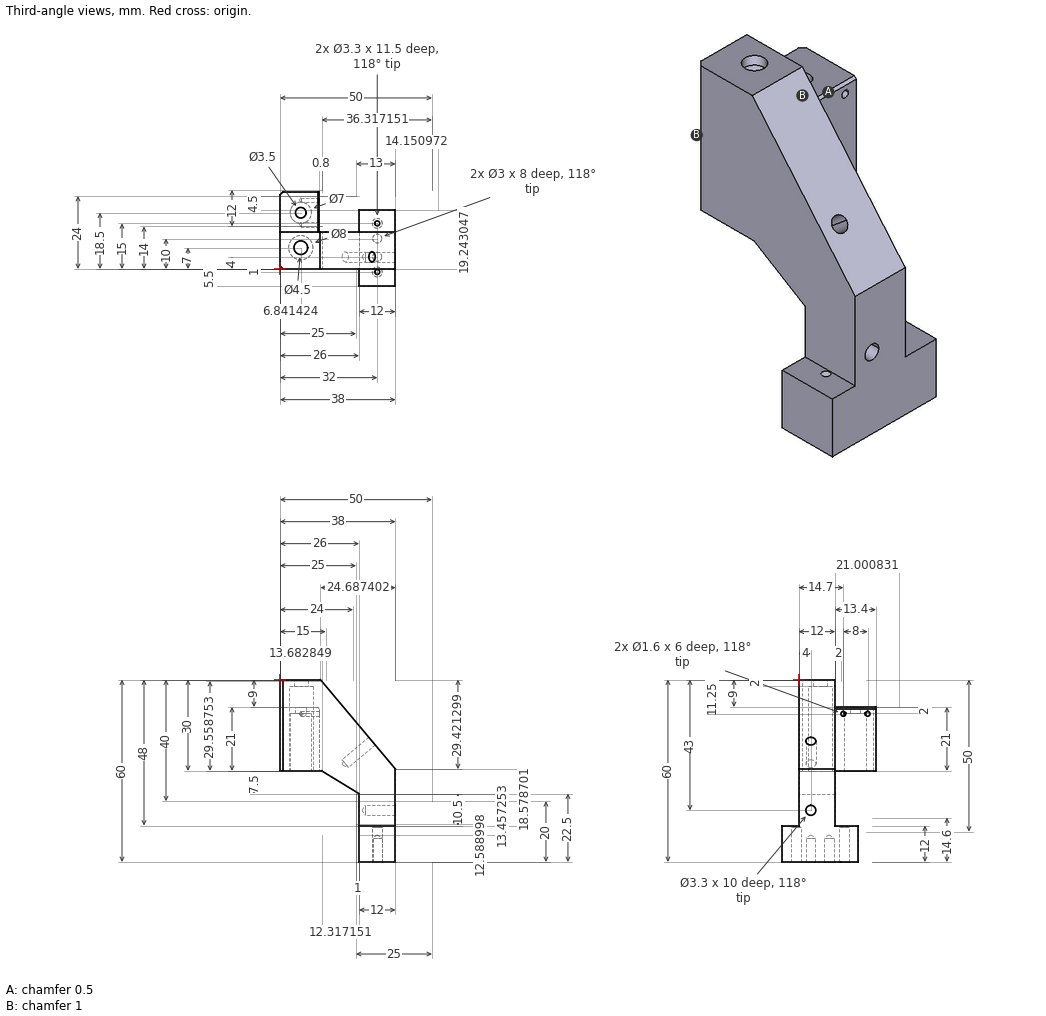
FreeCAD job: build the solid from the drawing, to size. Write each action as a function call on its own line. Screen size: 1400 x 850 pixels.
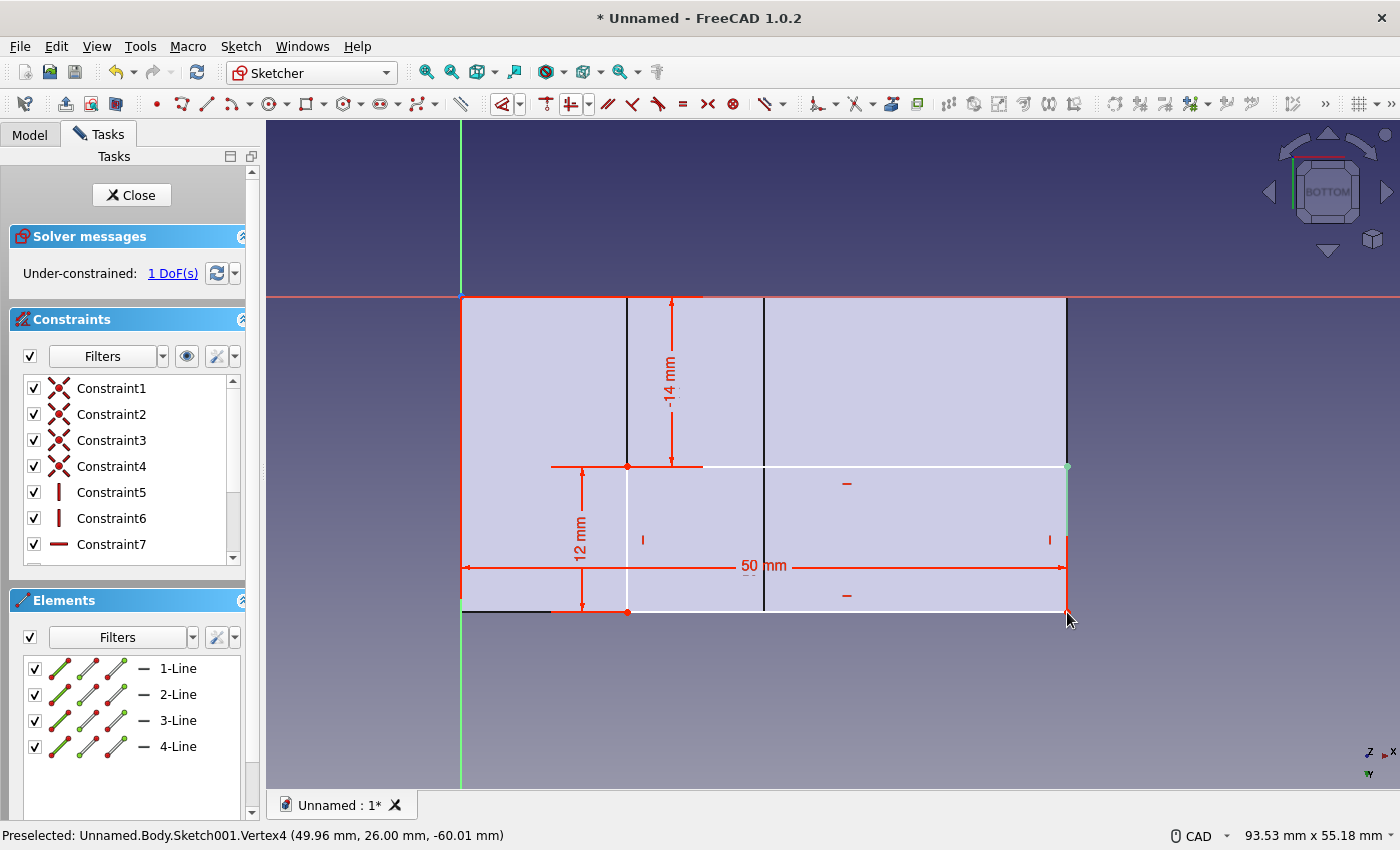
click(759, 612)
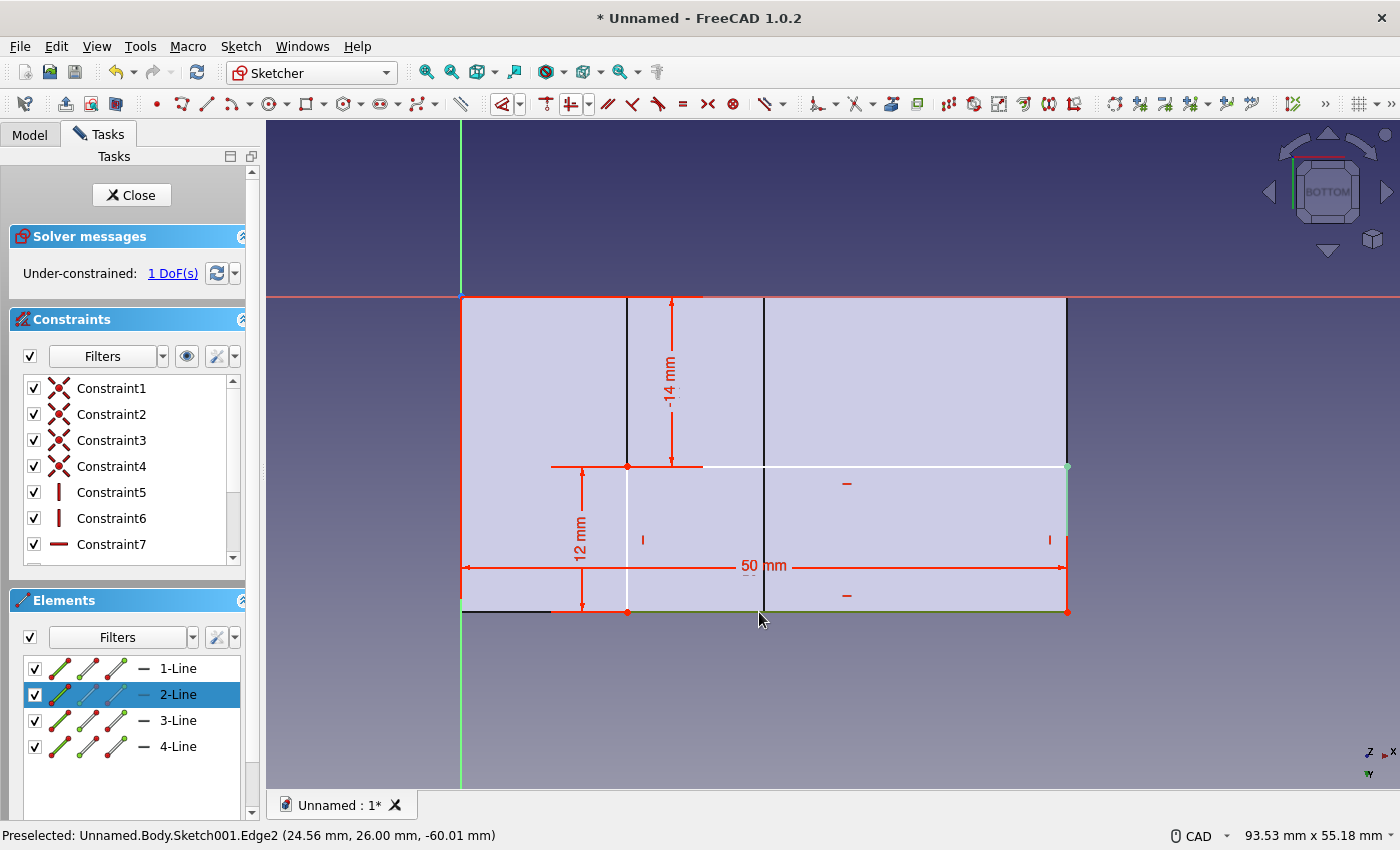
click(520, 104)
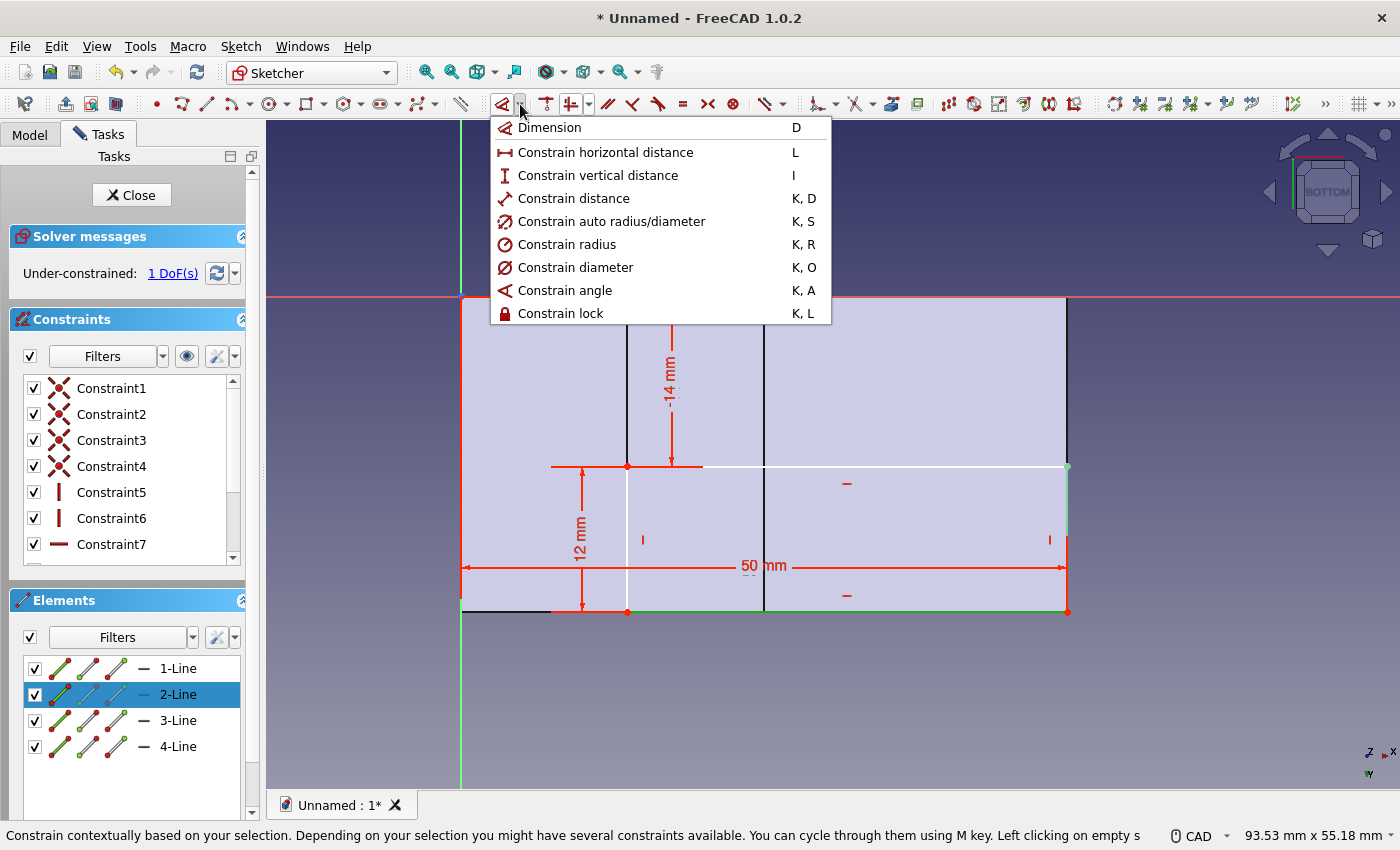
click(661, 152)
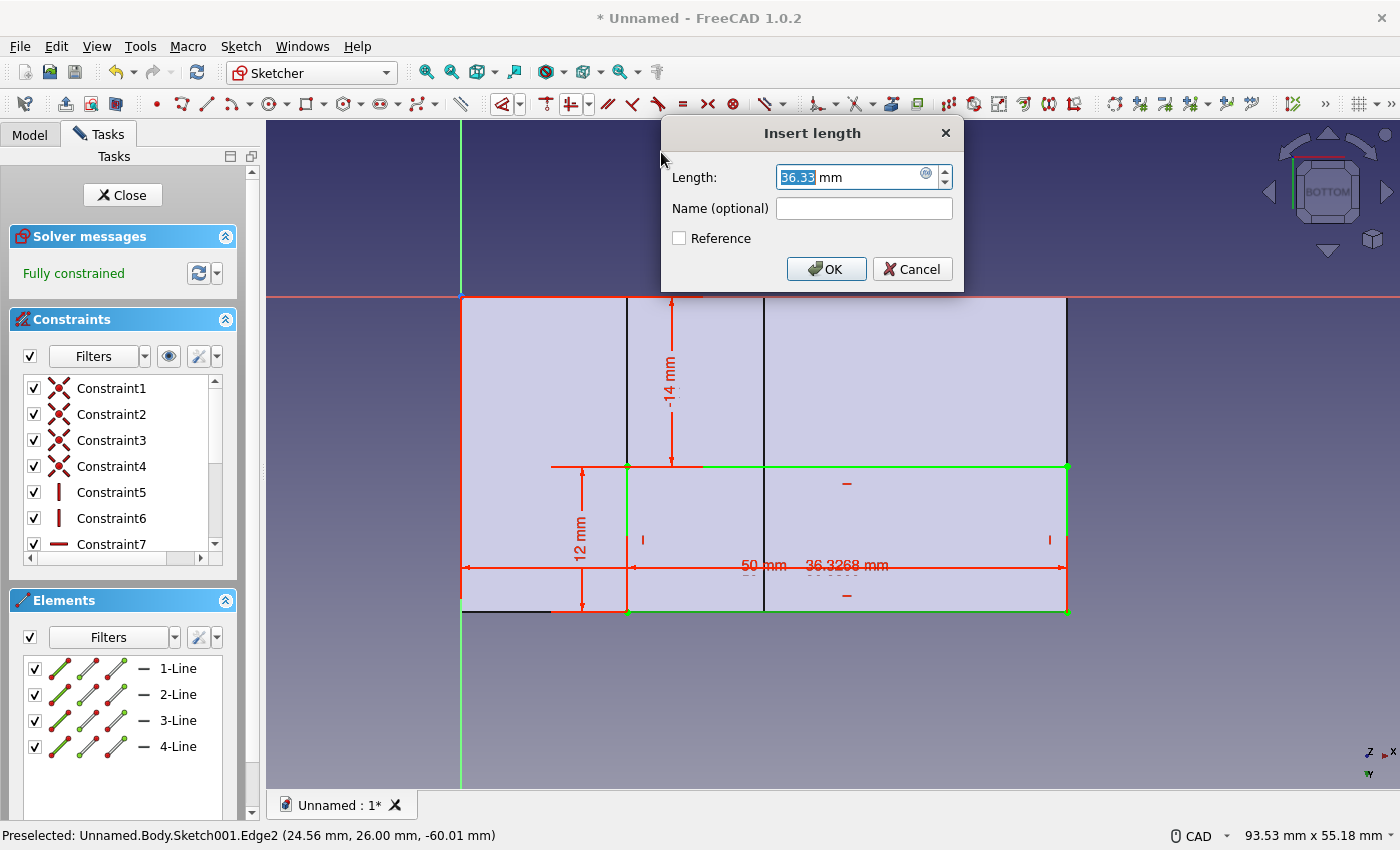
text(36.317151)
key(Return)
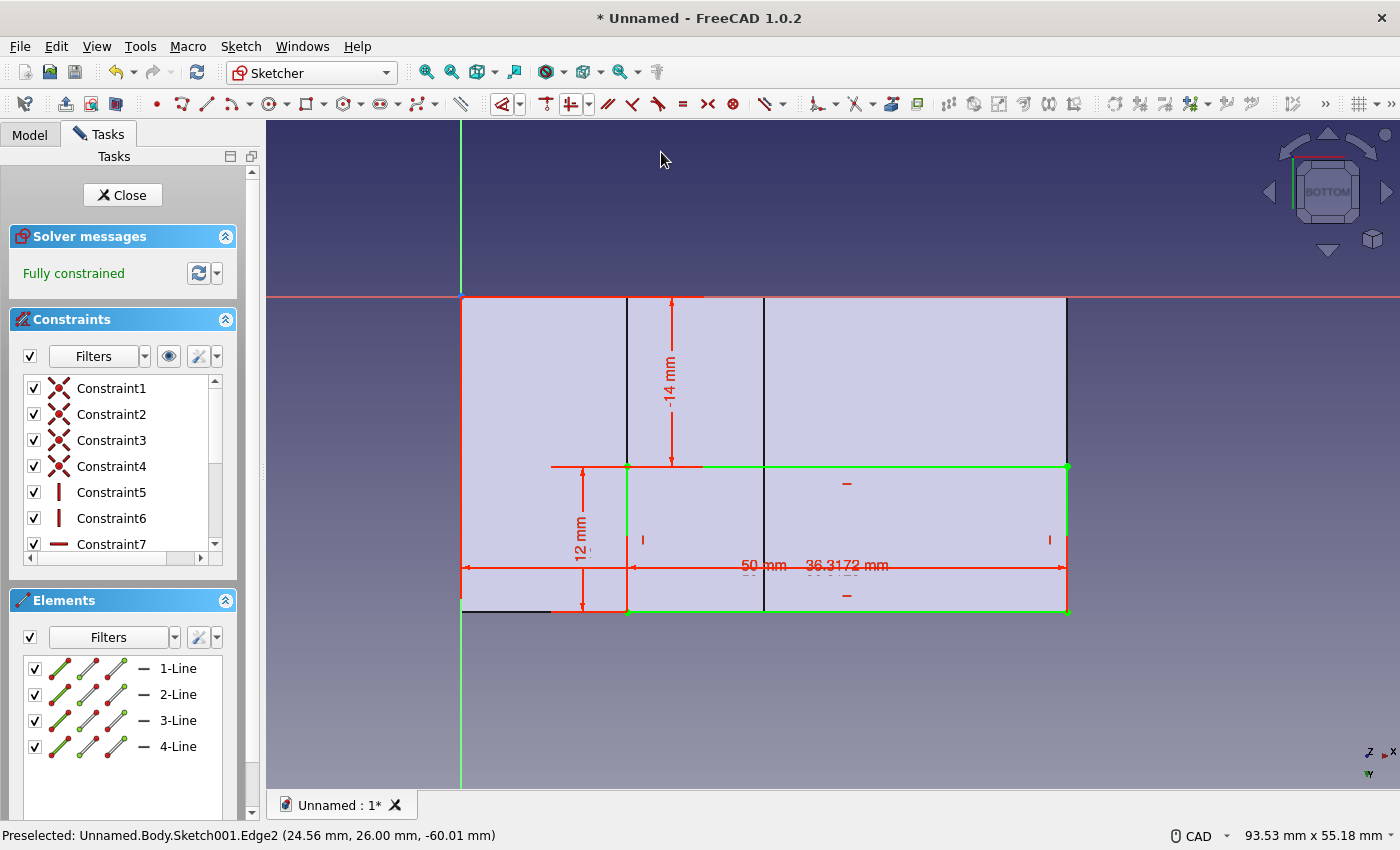
click(123, 195)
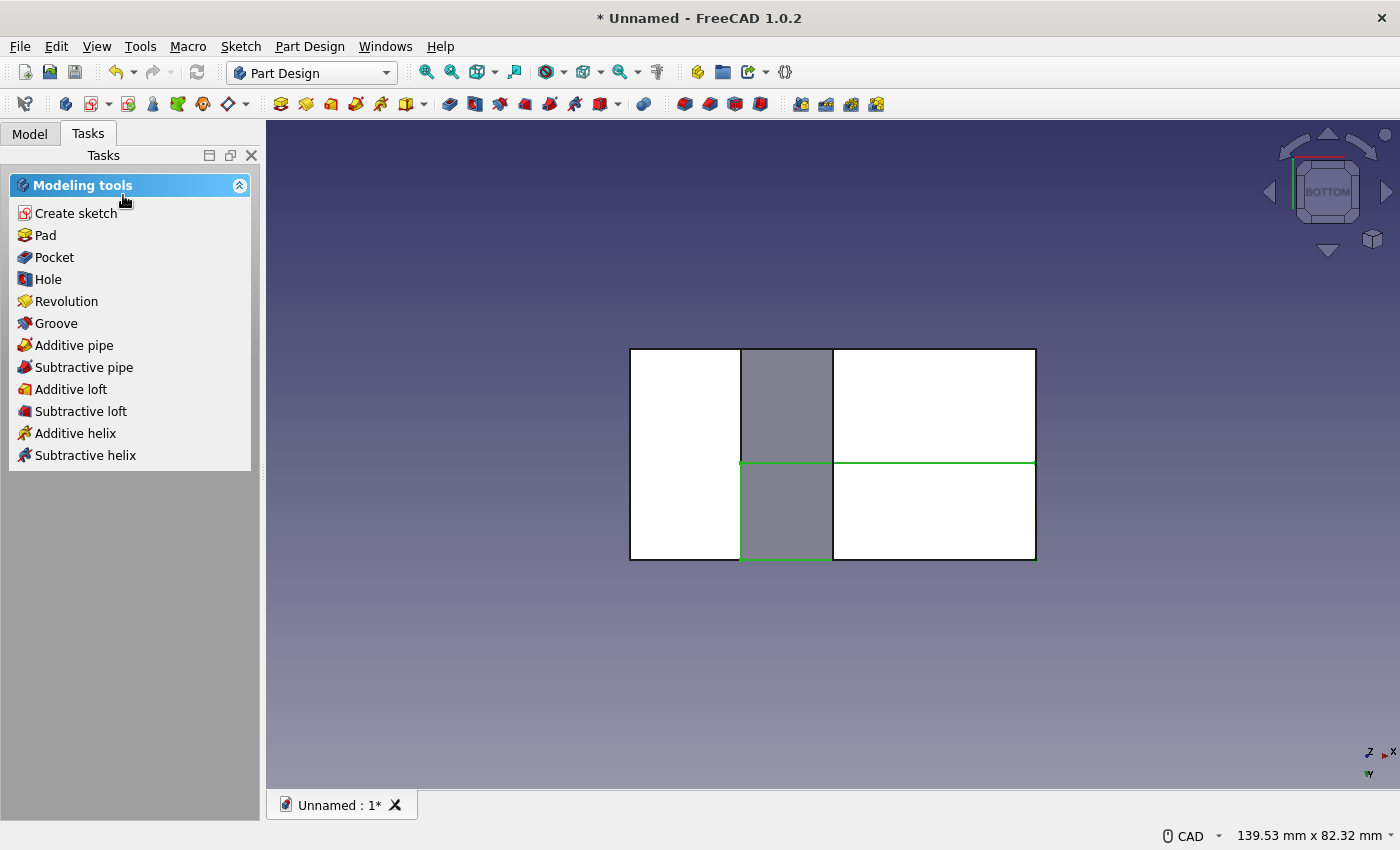
click(450, 104)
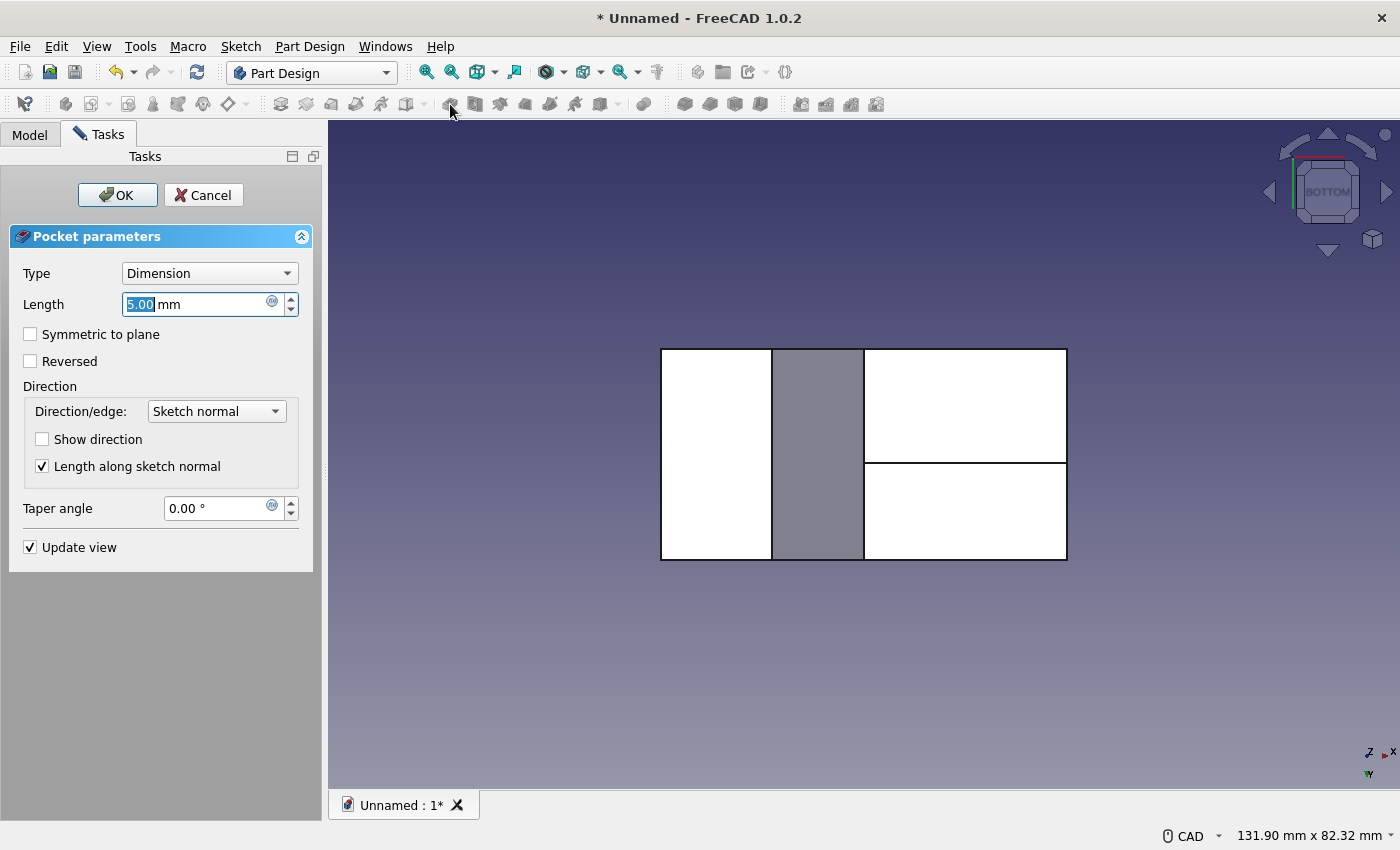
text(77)
key(Tab)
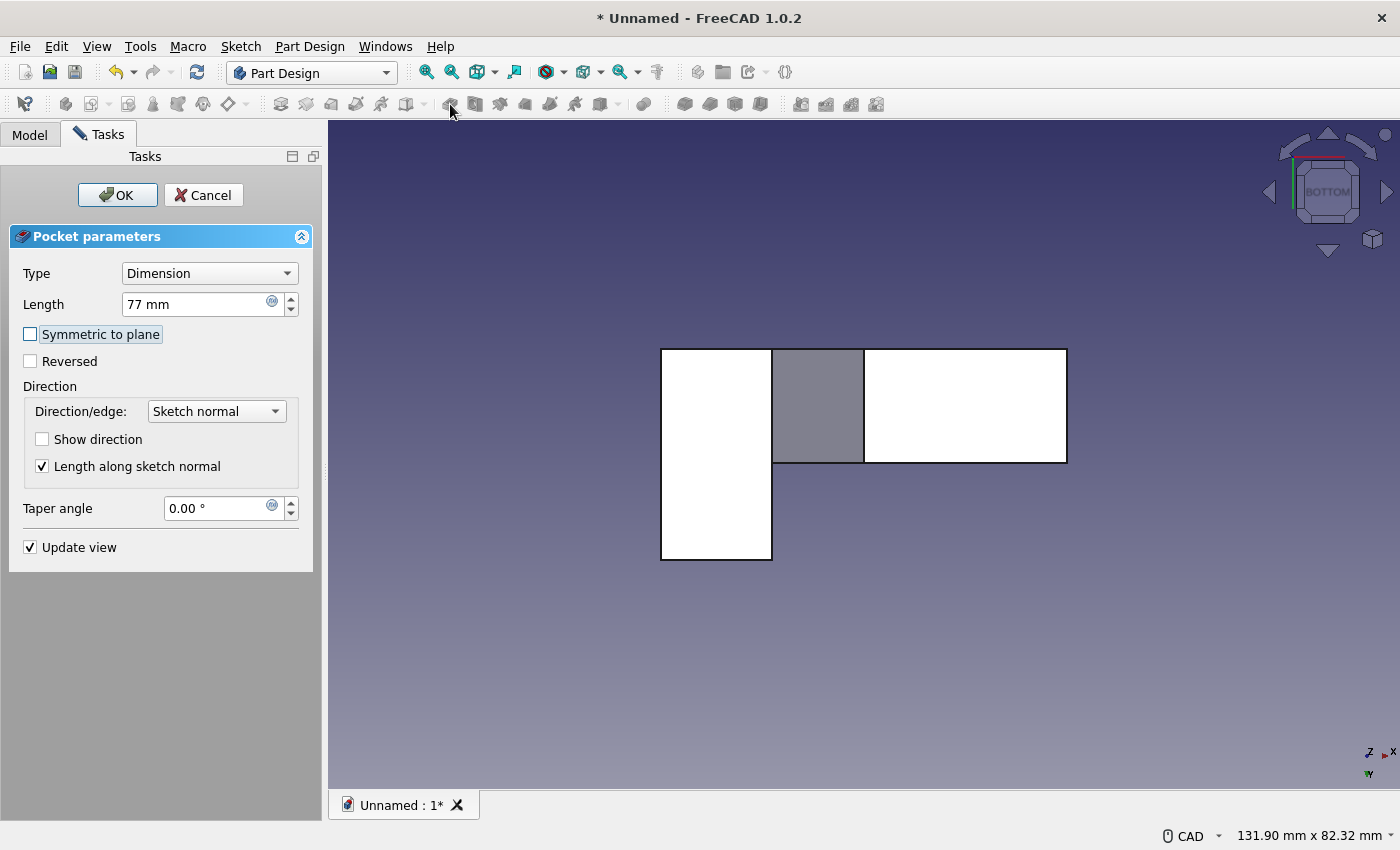
click(118, 195)